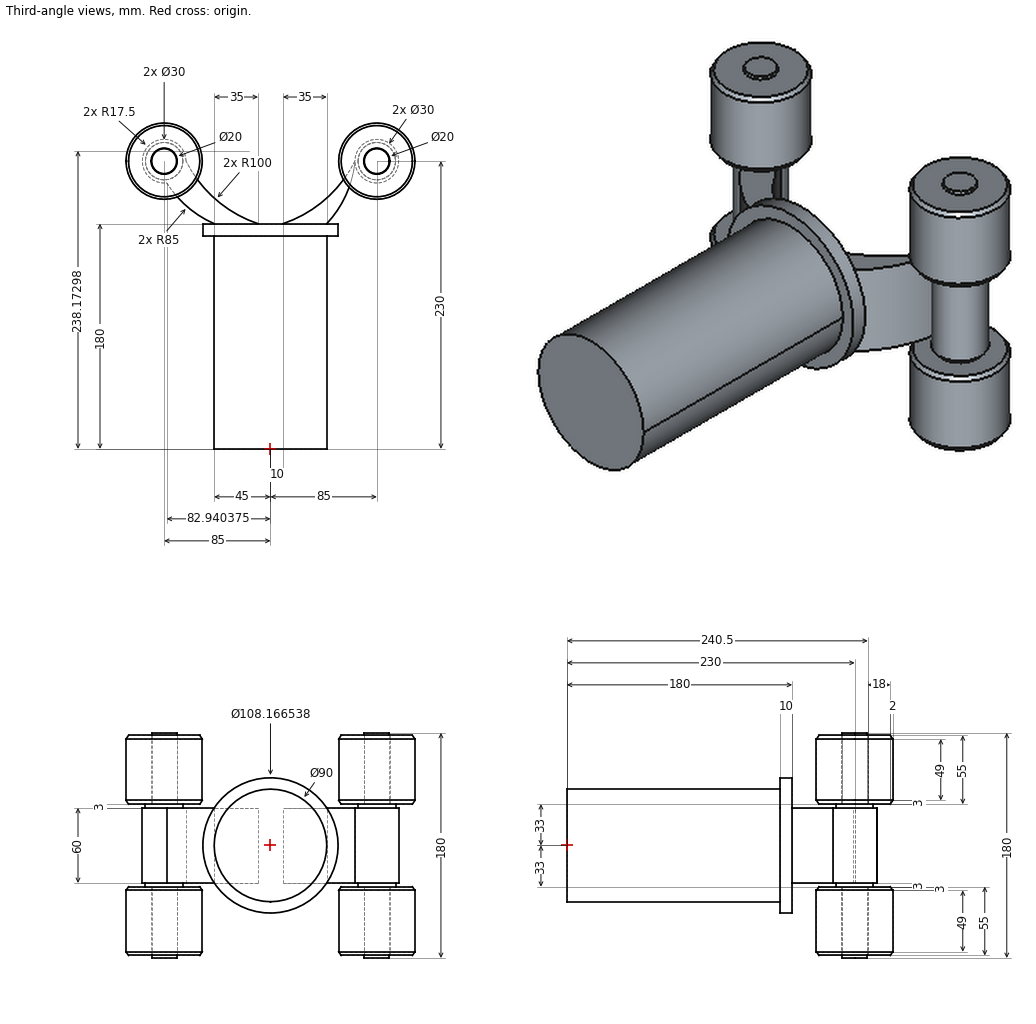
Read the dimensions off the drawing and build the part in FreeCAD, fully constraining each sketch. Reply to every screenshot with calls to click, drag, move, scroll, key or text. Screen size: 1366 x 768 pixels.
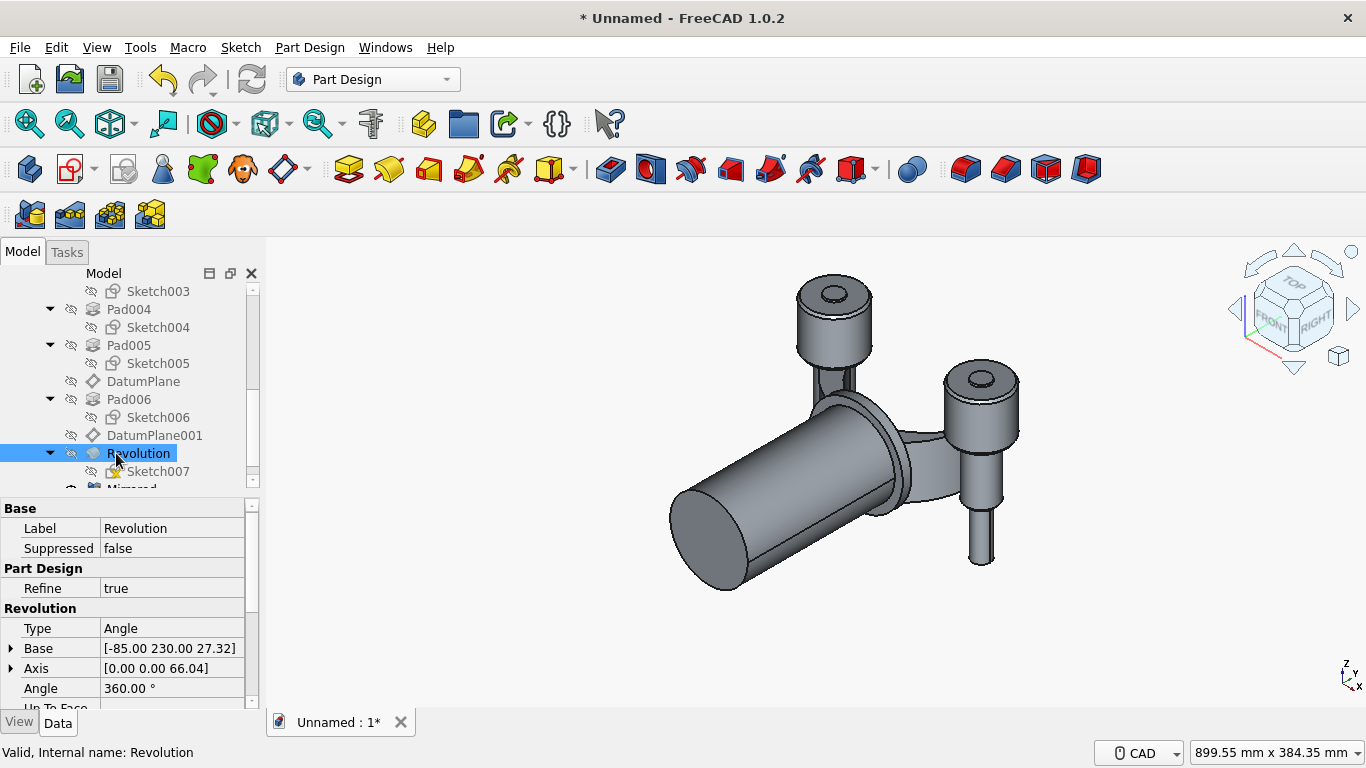
click(30, 214)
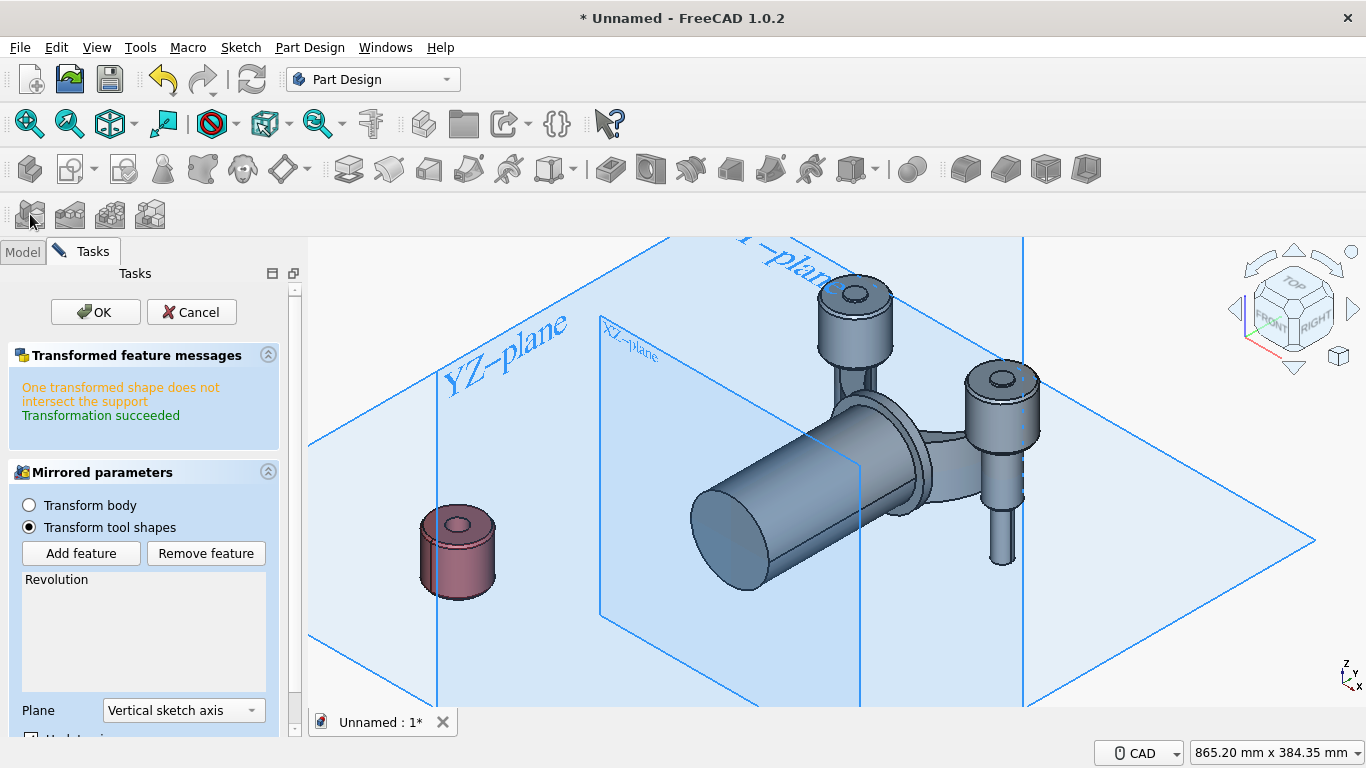
click(184, 710)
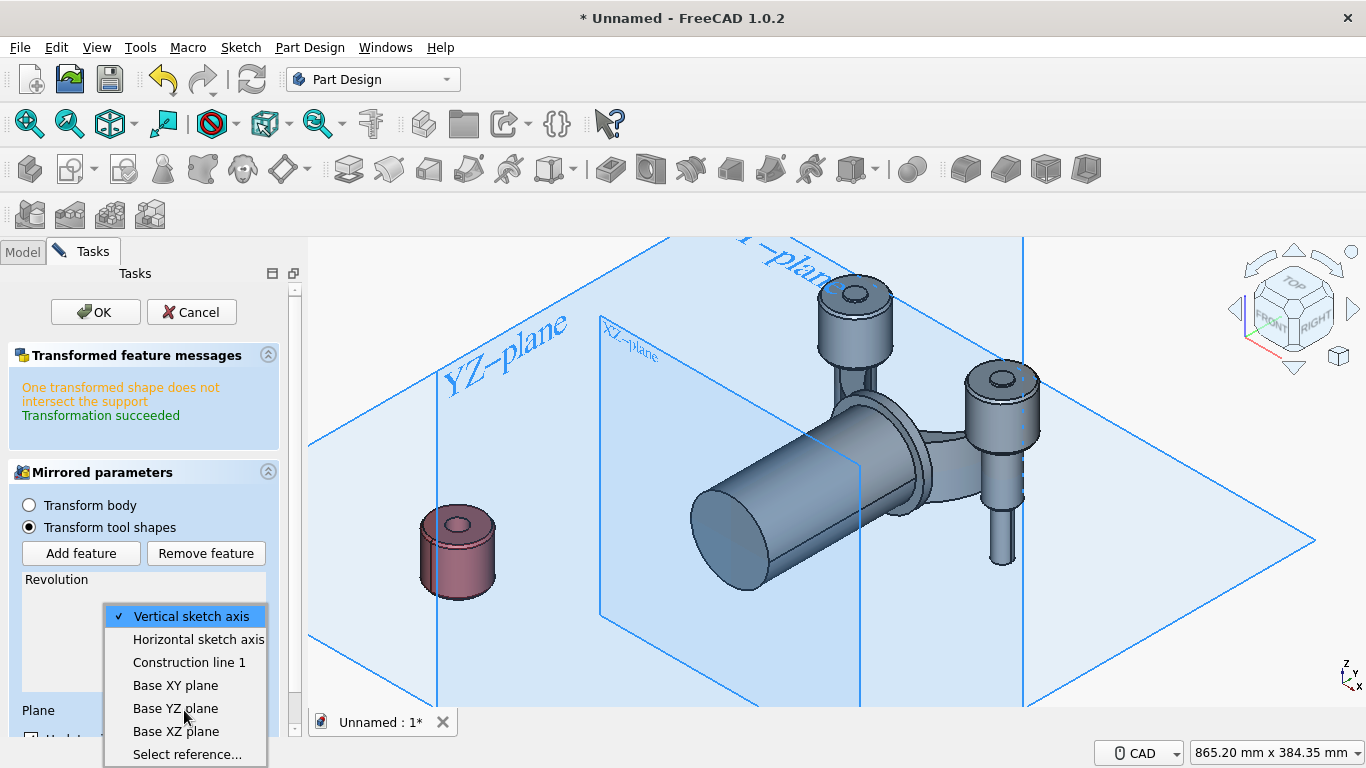
click(184, 686)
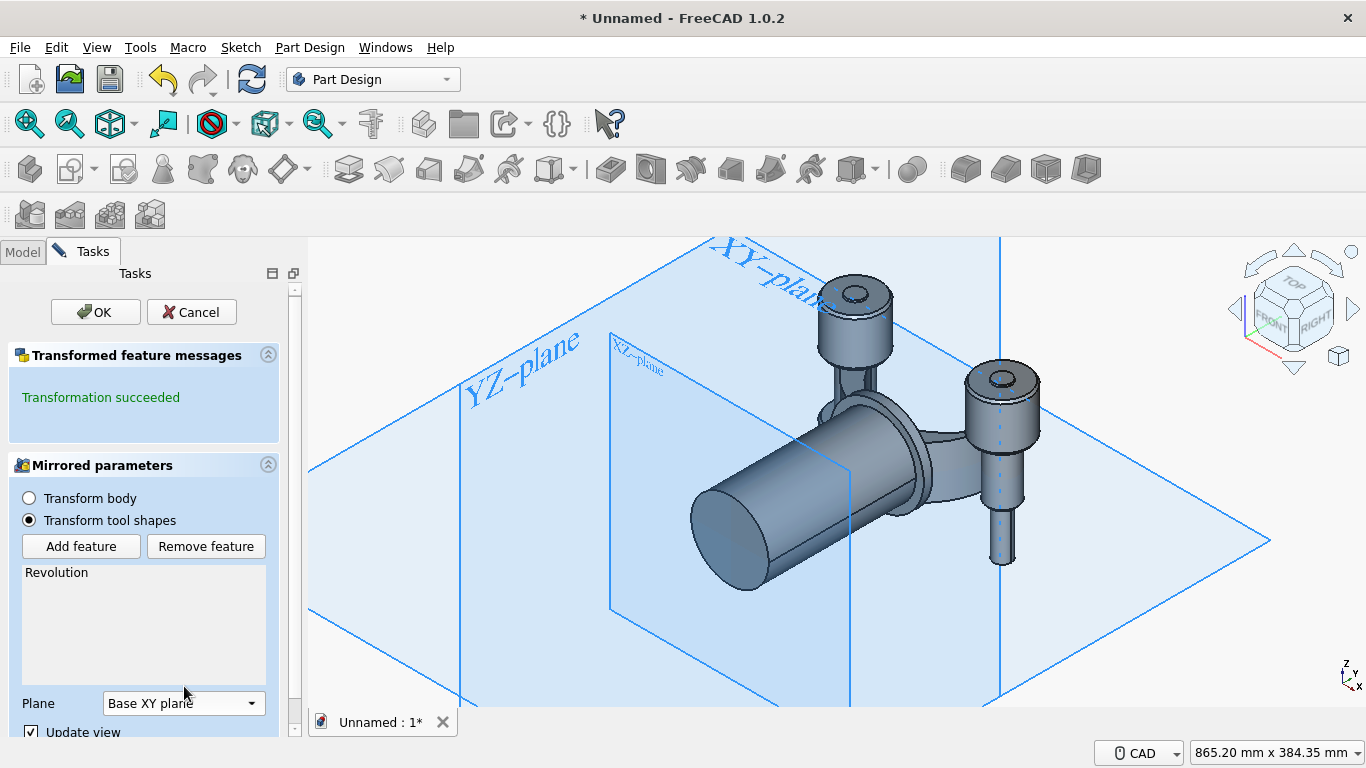
click(96, 312)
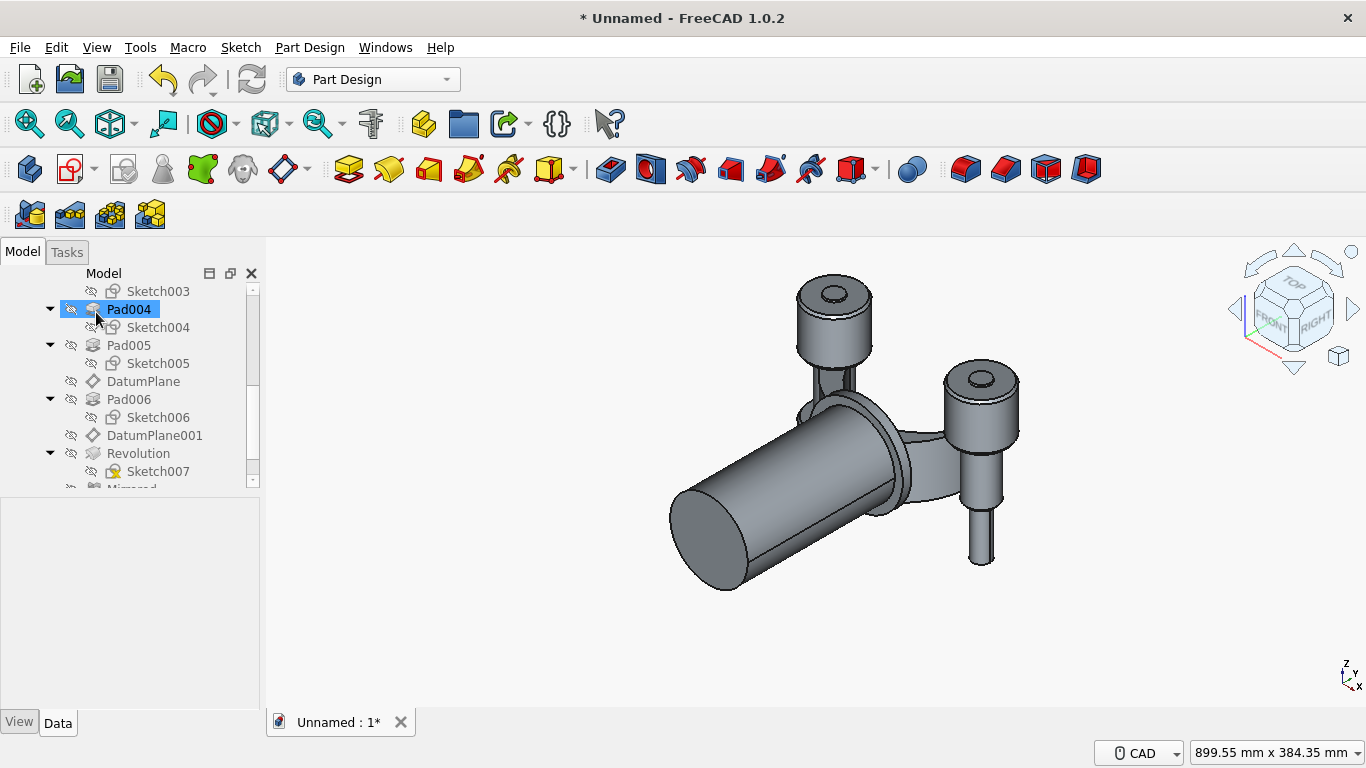
scroll(160, 377, down, 3)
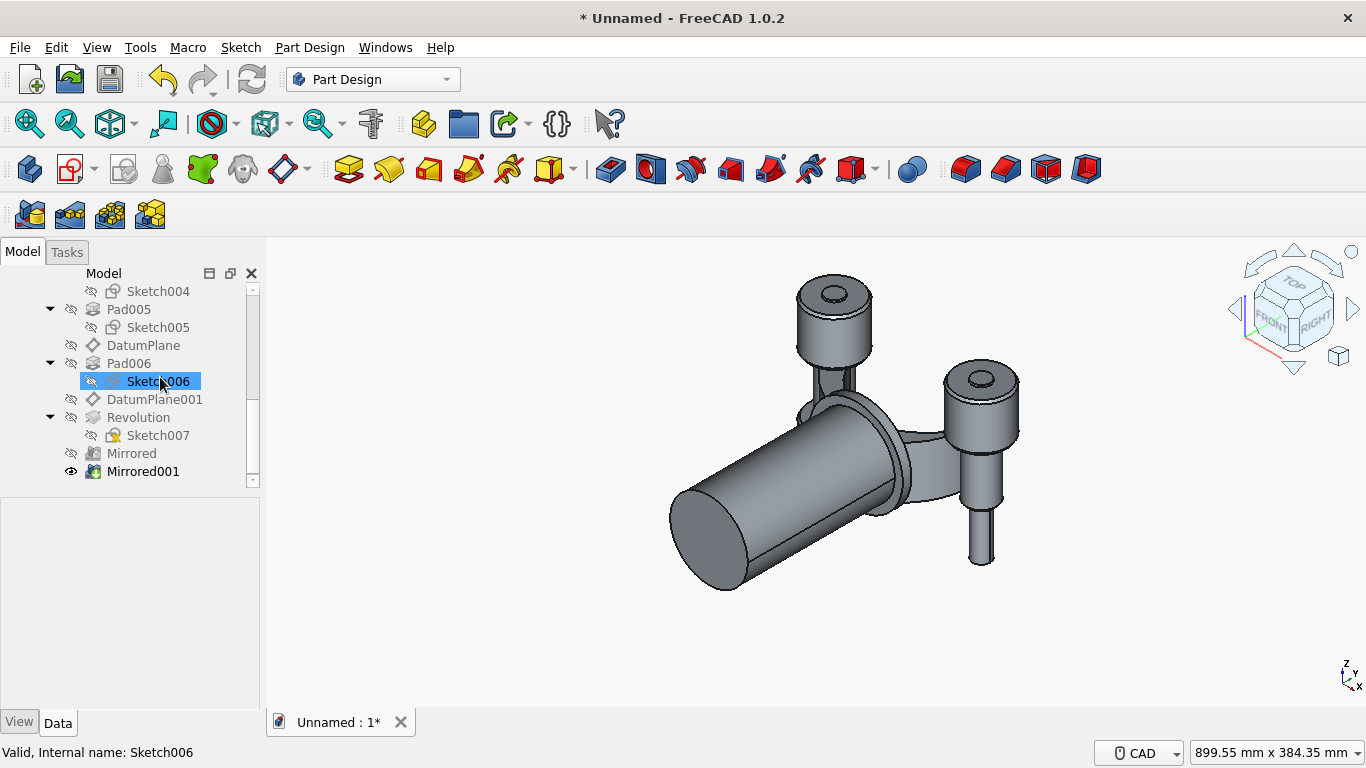
scroll(160, 377, up, 15)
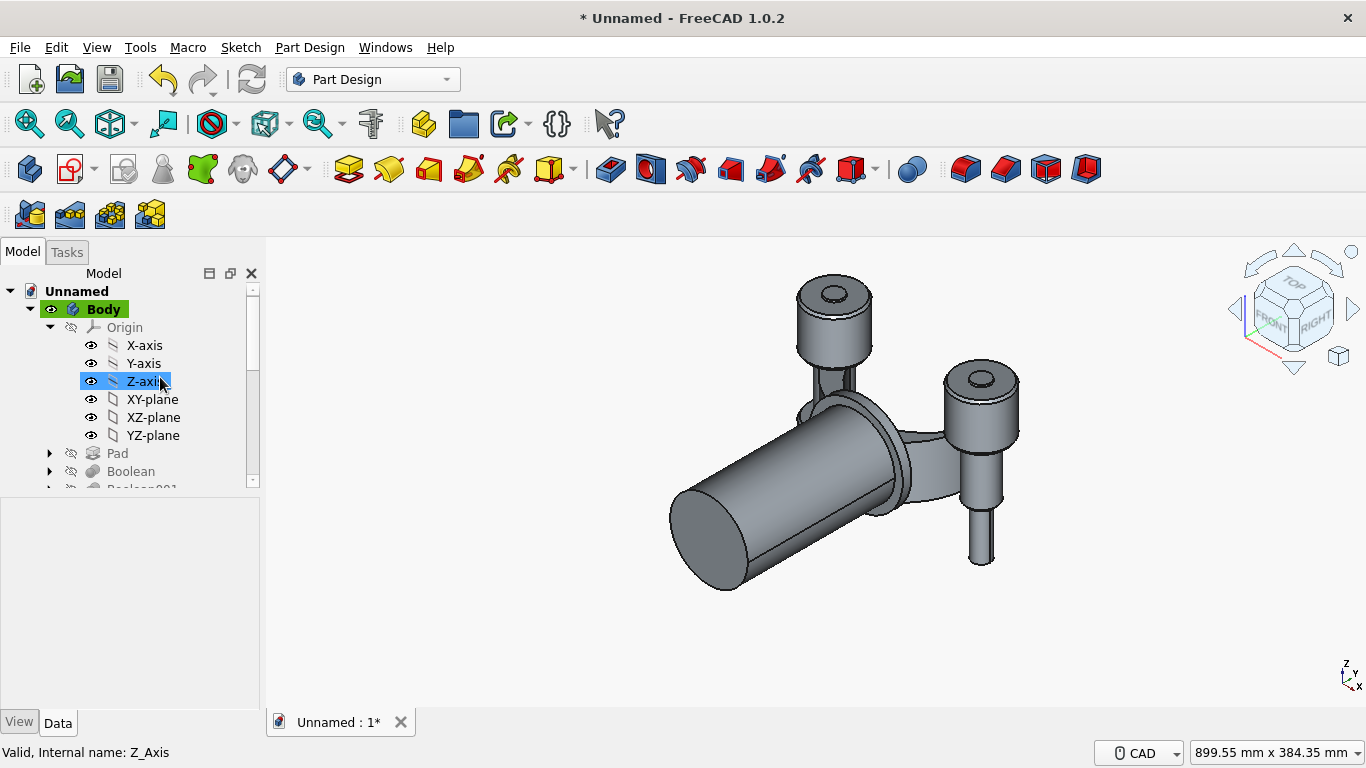
click(136, 435)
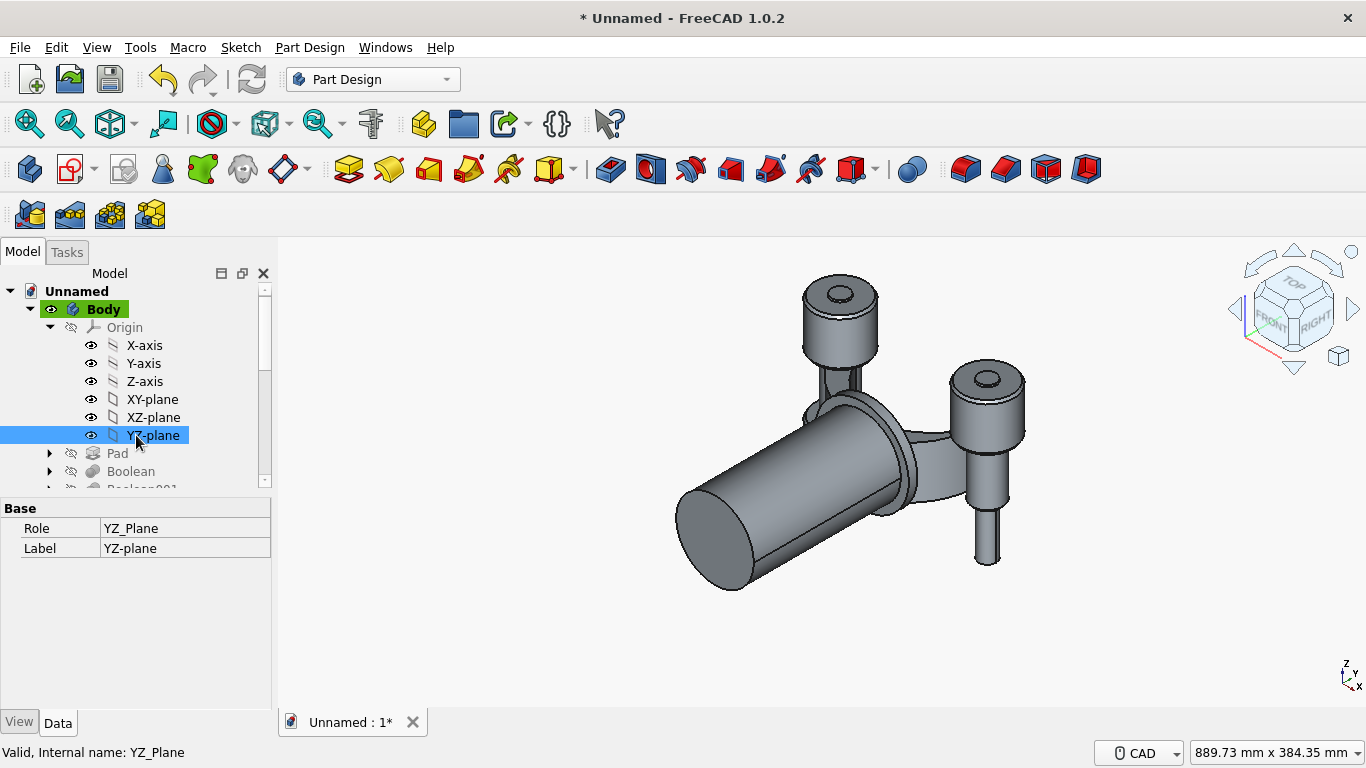
click(284, 170)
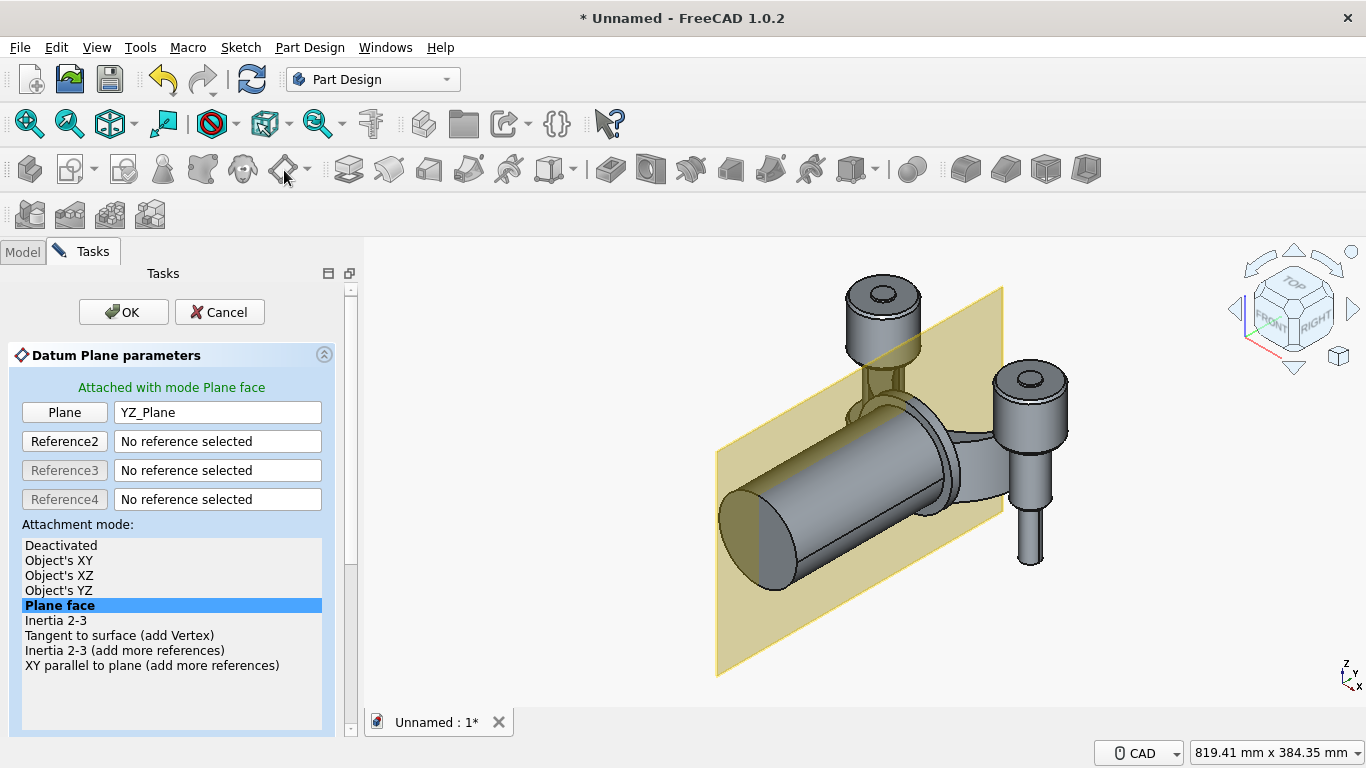
scroll(351, 510, down, 3)